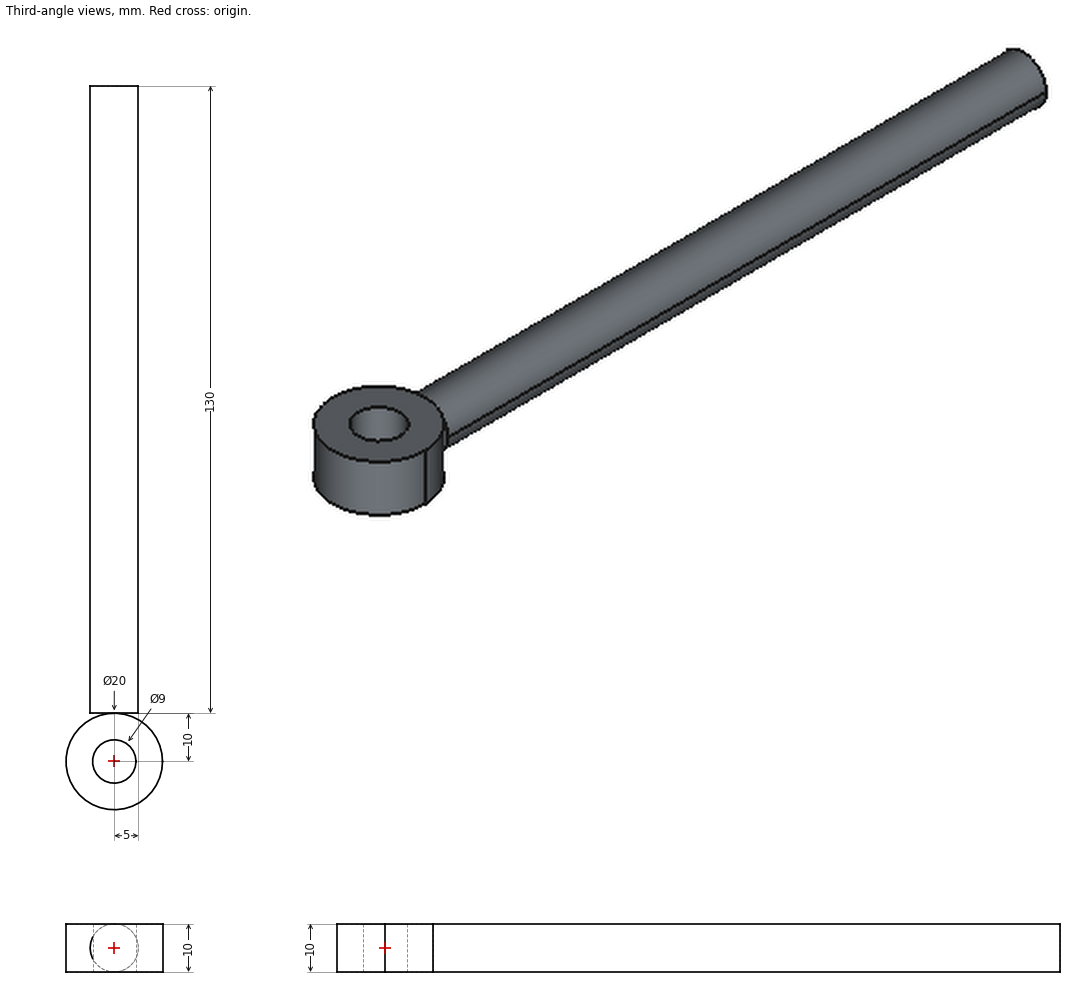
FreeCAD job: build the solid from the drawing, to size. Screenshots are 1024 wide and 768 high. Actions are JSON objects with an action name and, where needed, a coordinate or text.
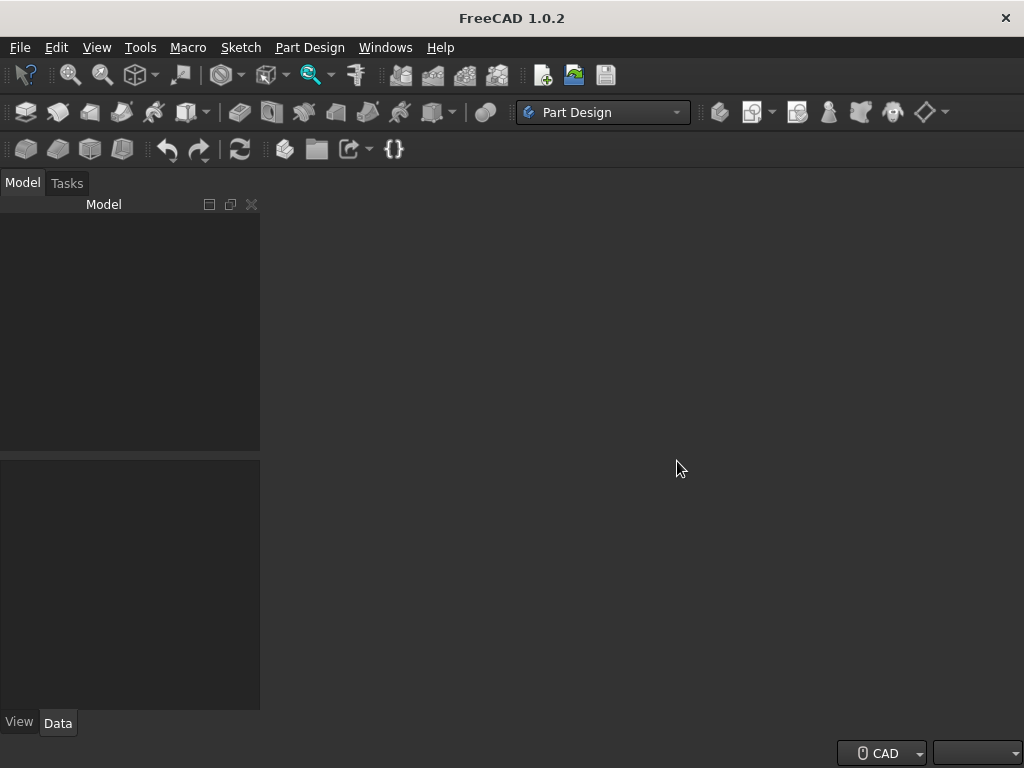
{"action": "left_click", "coordinate": [542, 76]}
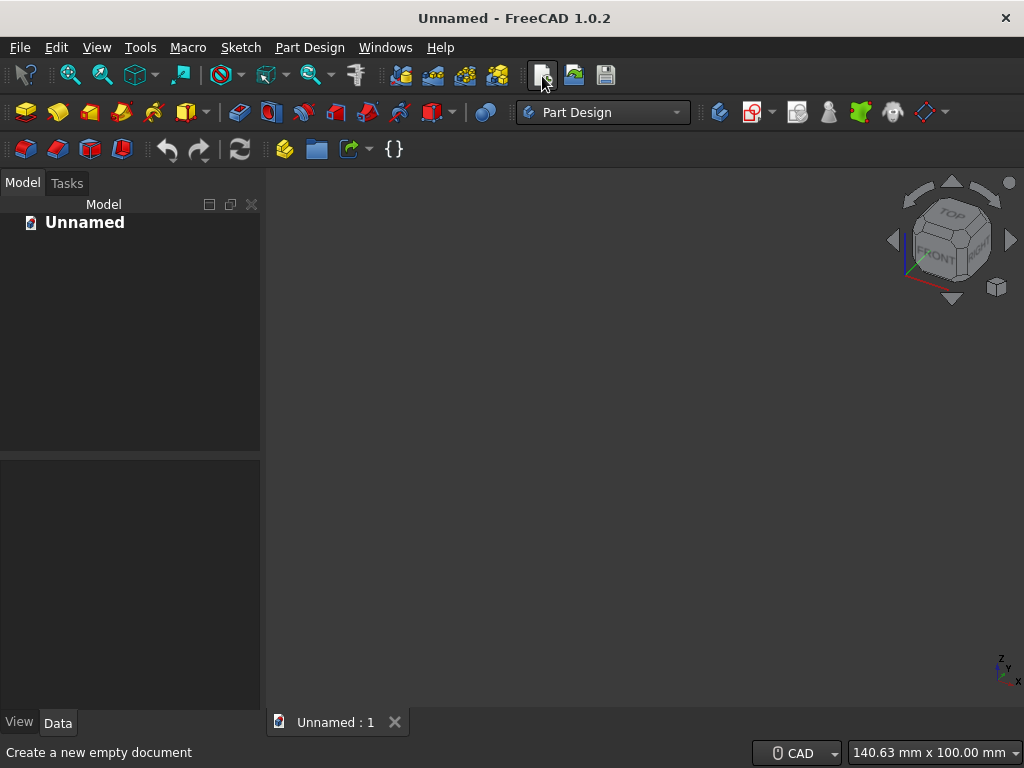
{"action": "left_click", "coordinate": [752, 112]}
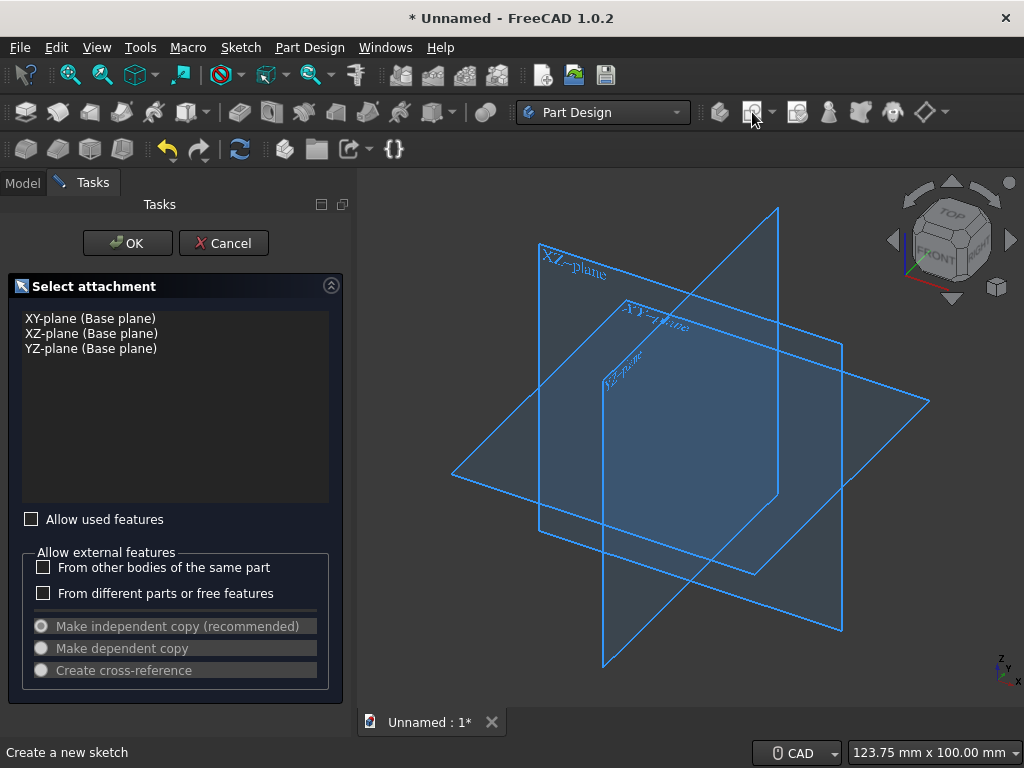
{"action": "left_click", "coordinate": [82, 318]}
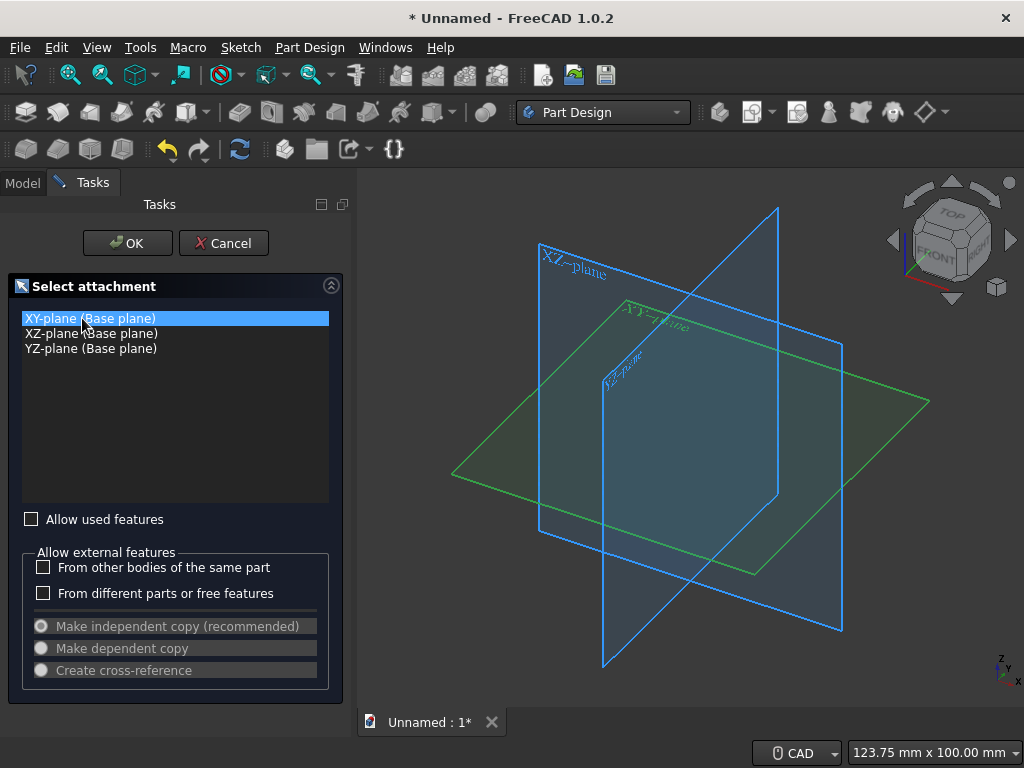
{"action": "left_click", "coordinate": [128, 243]}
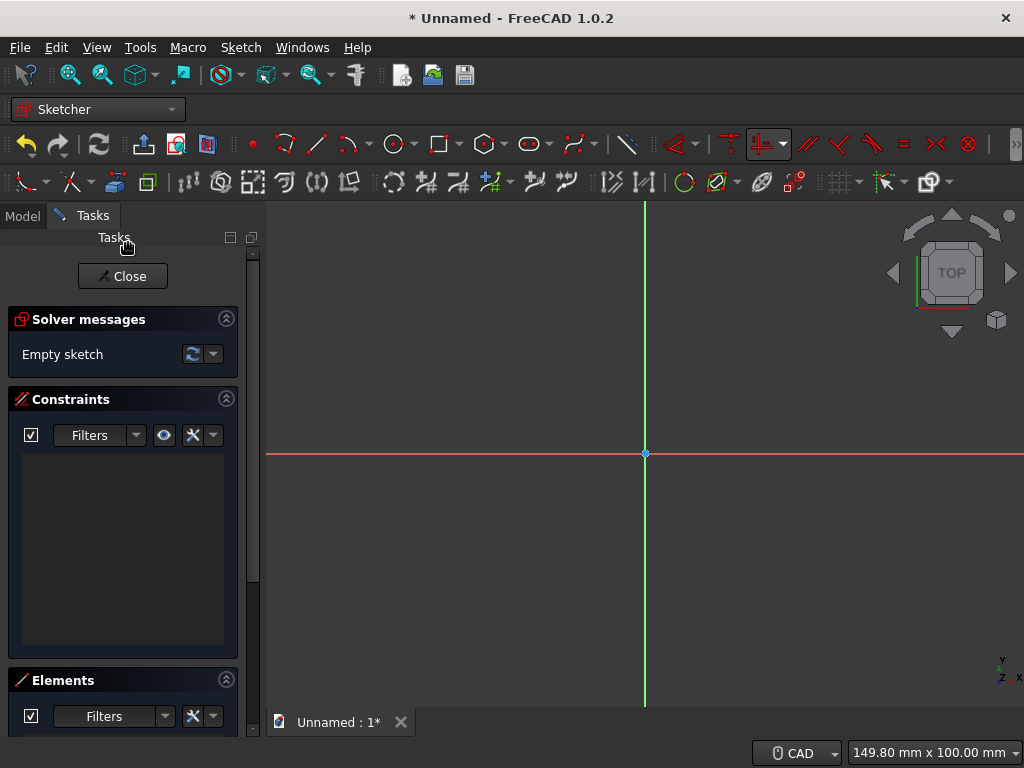
{"action": "scroll", "coordinate": [675, 454], "scroll_direction": "up", "scroll_amount": 6}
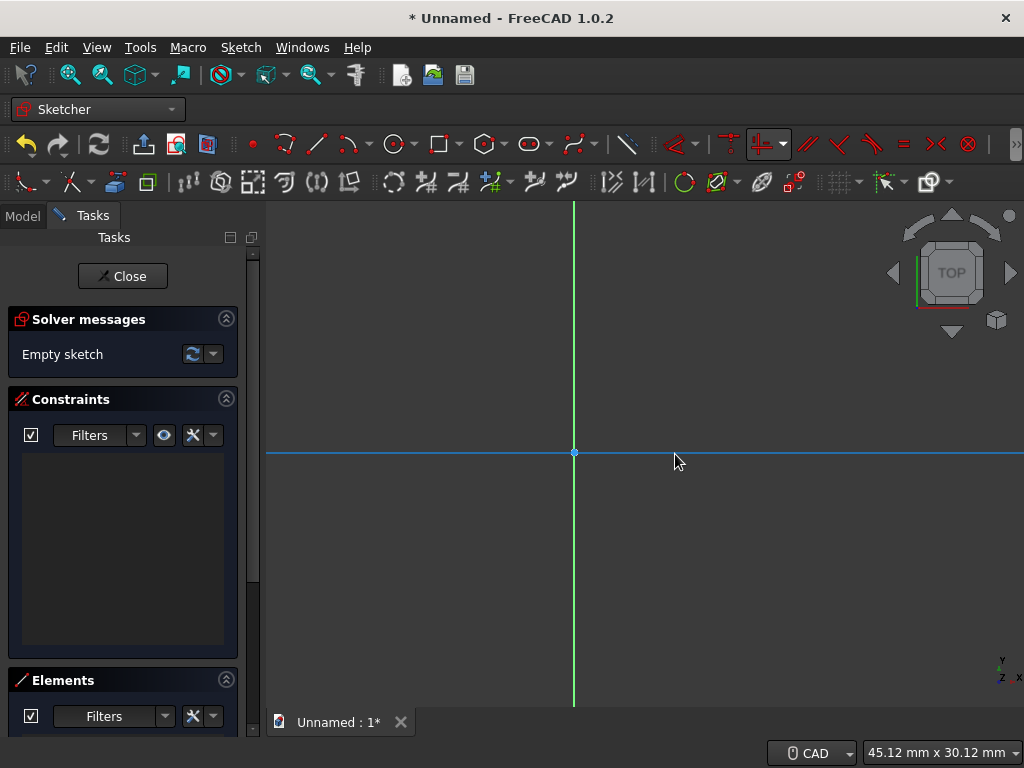
{"action": "left_click", "coordinate": [394, 144]}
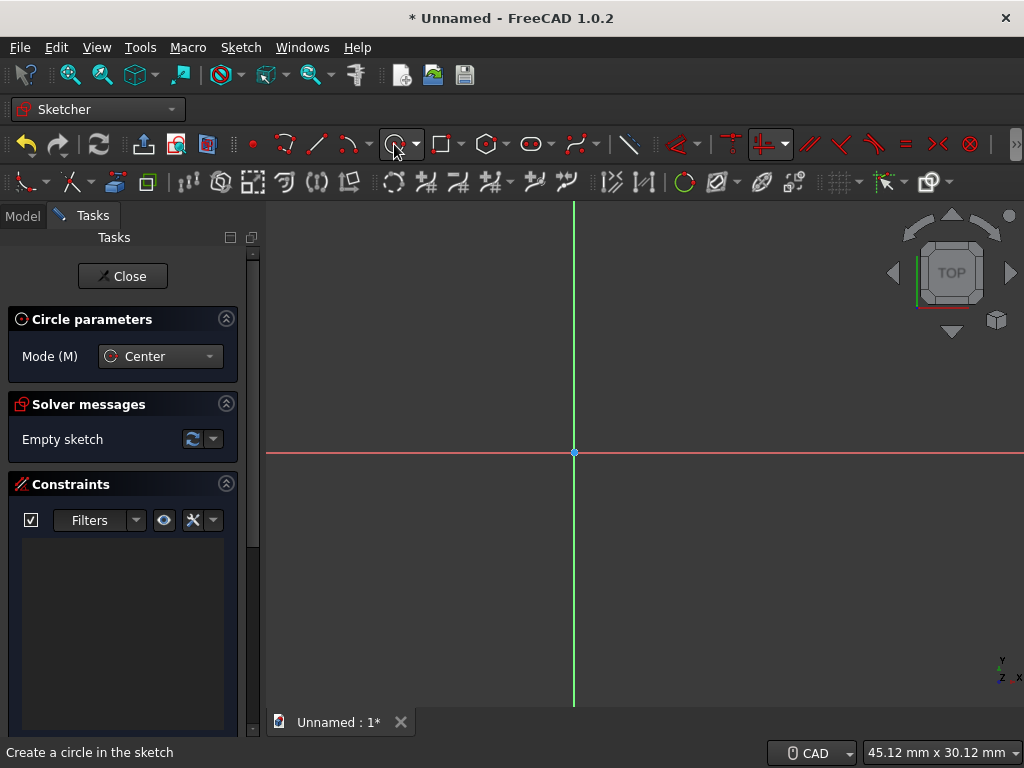
{"action": "left_click", "coordinate": [574, 453]}
{"action": "left_click", "coordinate": [693, 334]}
{"action": "key", "text": "Escape"}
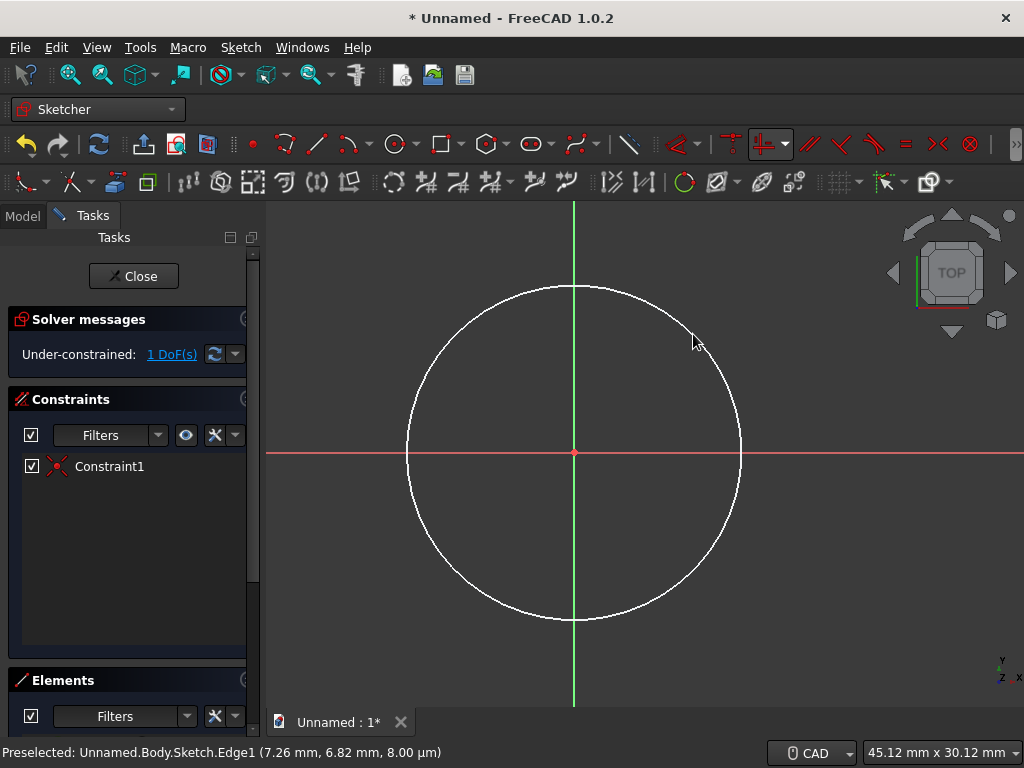
{"action": "left_click", "coordinate": [676, 144]}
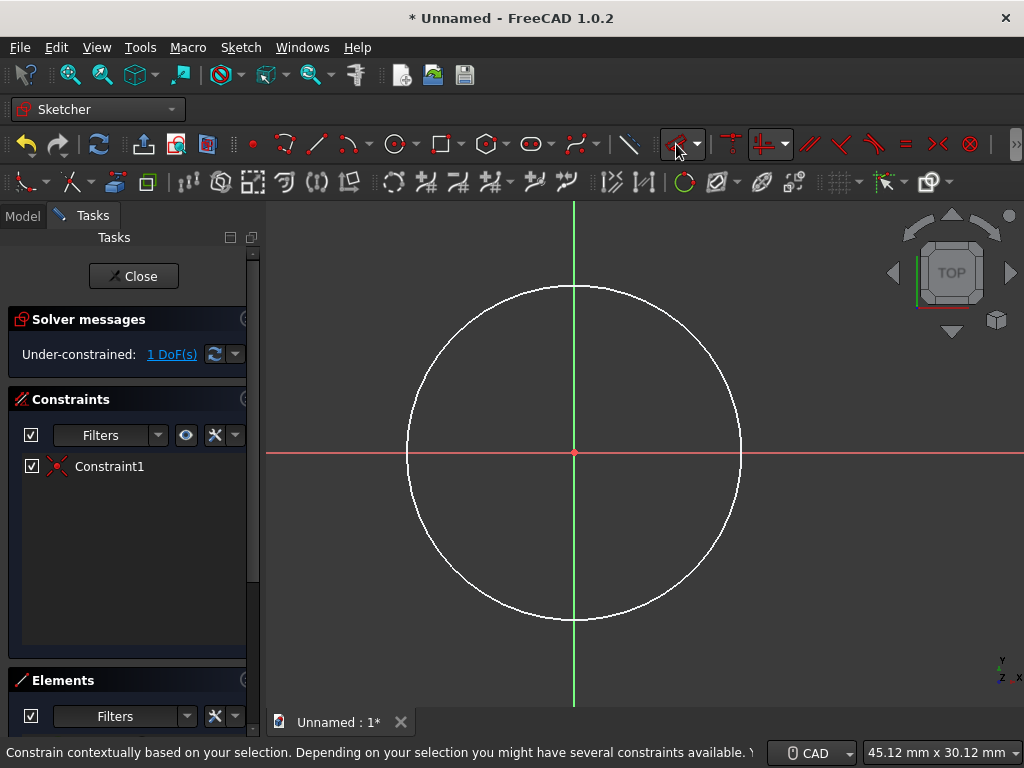
{"action": "left_click", "coordinate": [692, 334]}
{"action": "left_click", "coordinate": [715, 311]}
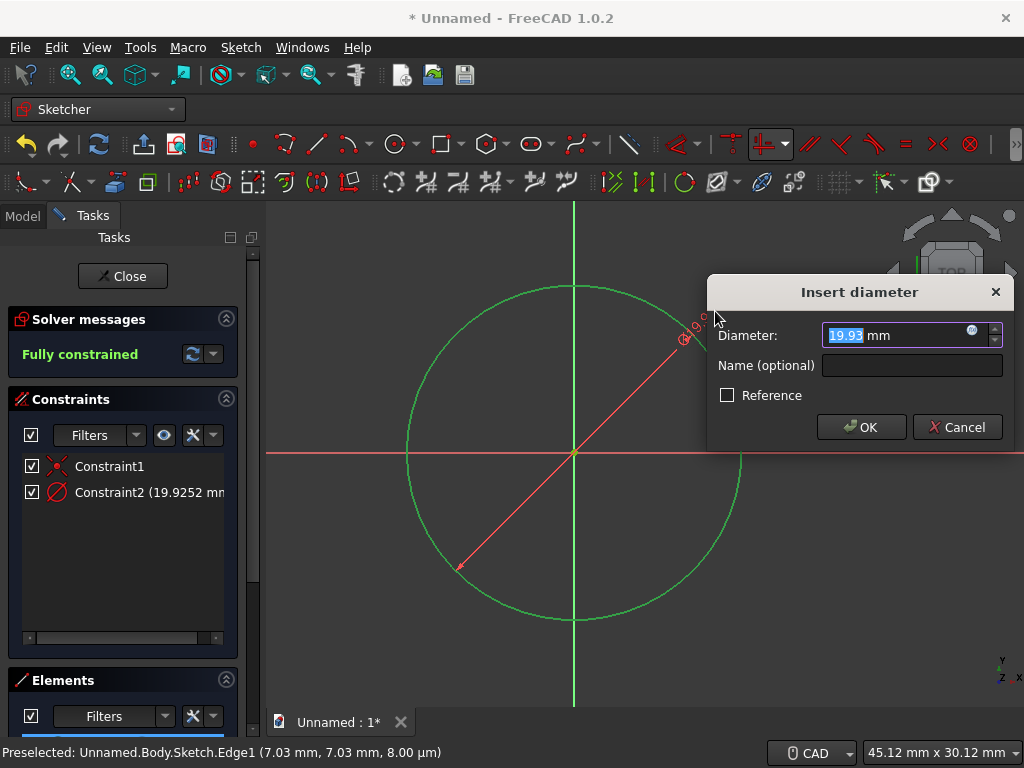
{"action": "type", "text": "20"}
{"action": "key", "text": "Return"}
{"action": "key", "text": "Escape"}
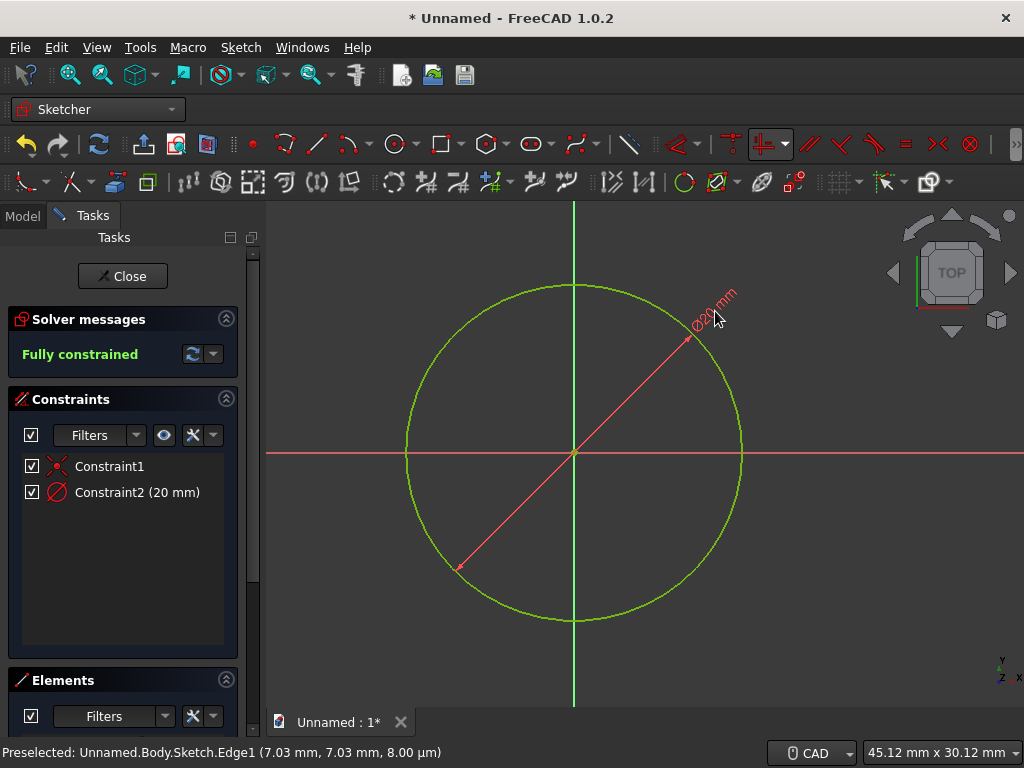
{"action": "left_click", "coordinate": [123, 276]}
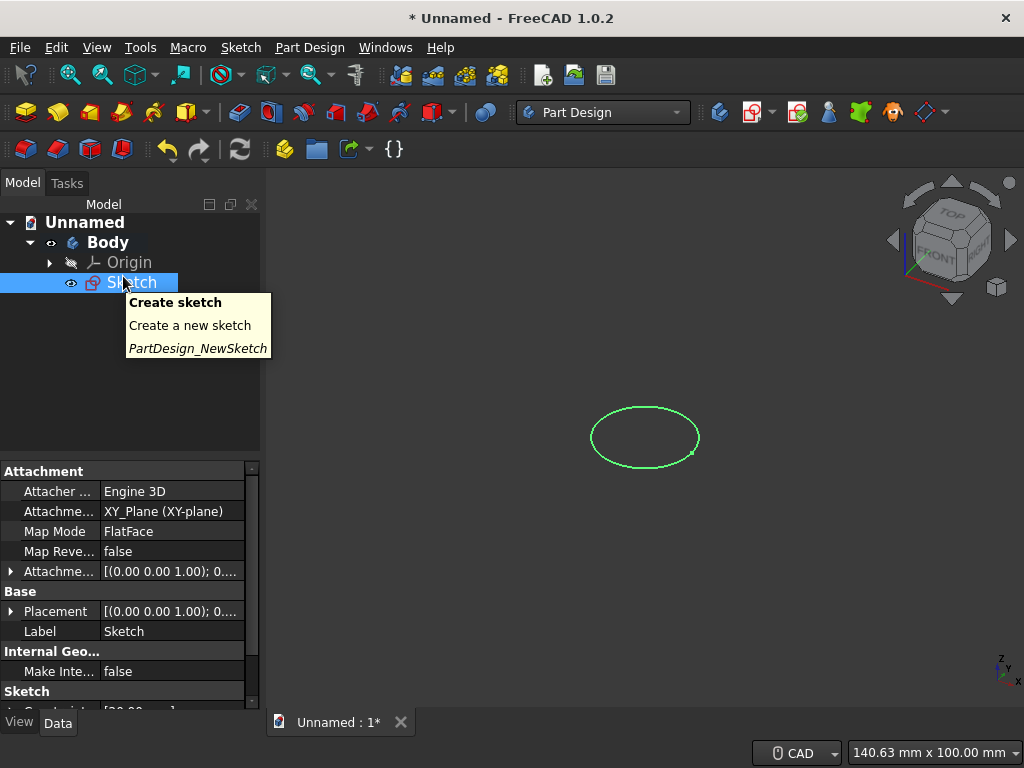
{"action": "left_click", "coordinate": [26, 112]}